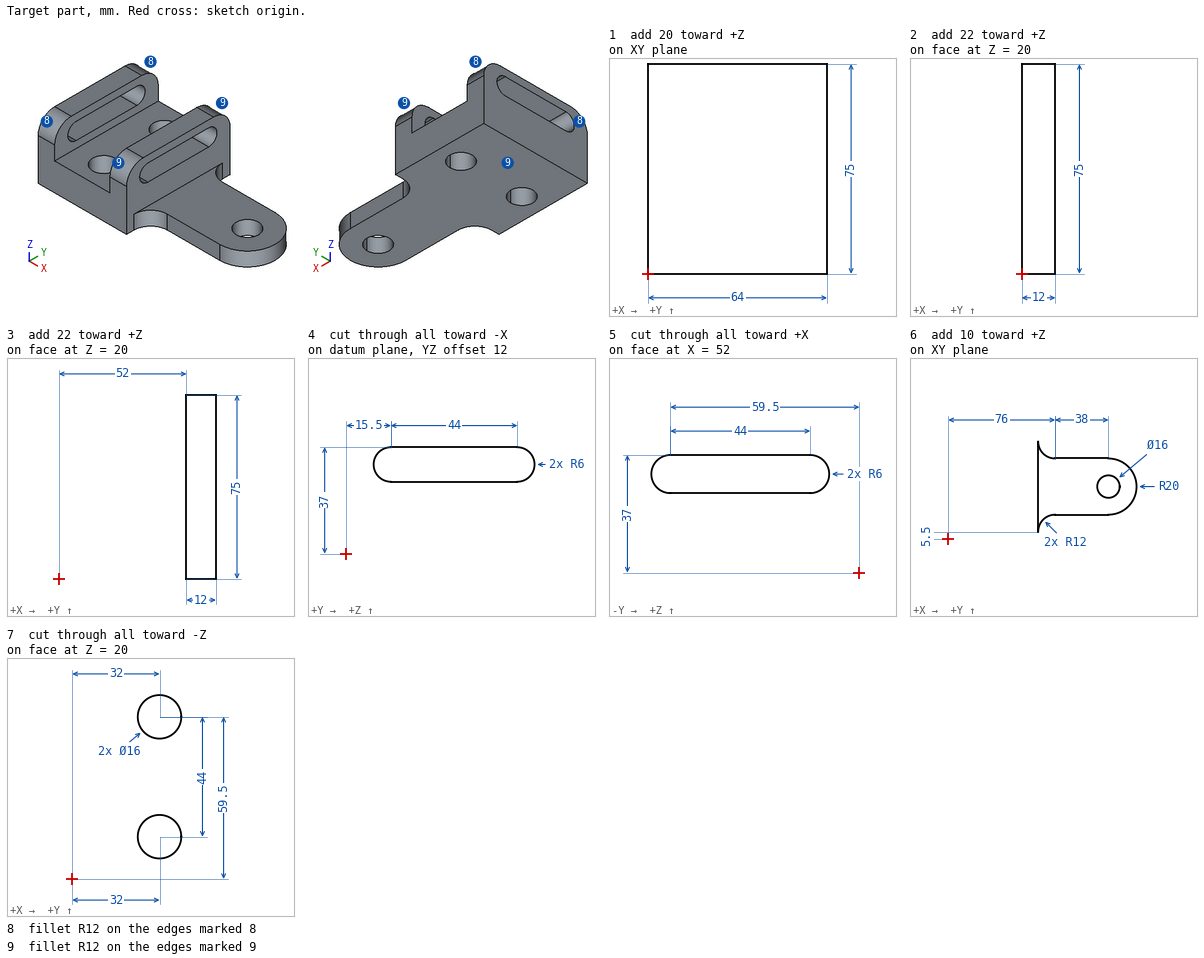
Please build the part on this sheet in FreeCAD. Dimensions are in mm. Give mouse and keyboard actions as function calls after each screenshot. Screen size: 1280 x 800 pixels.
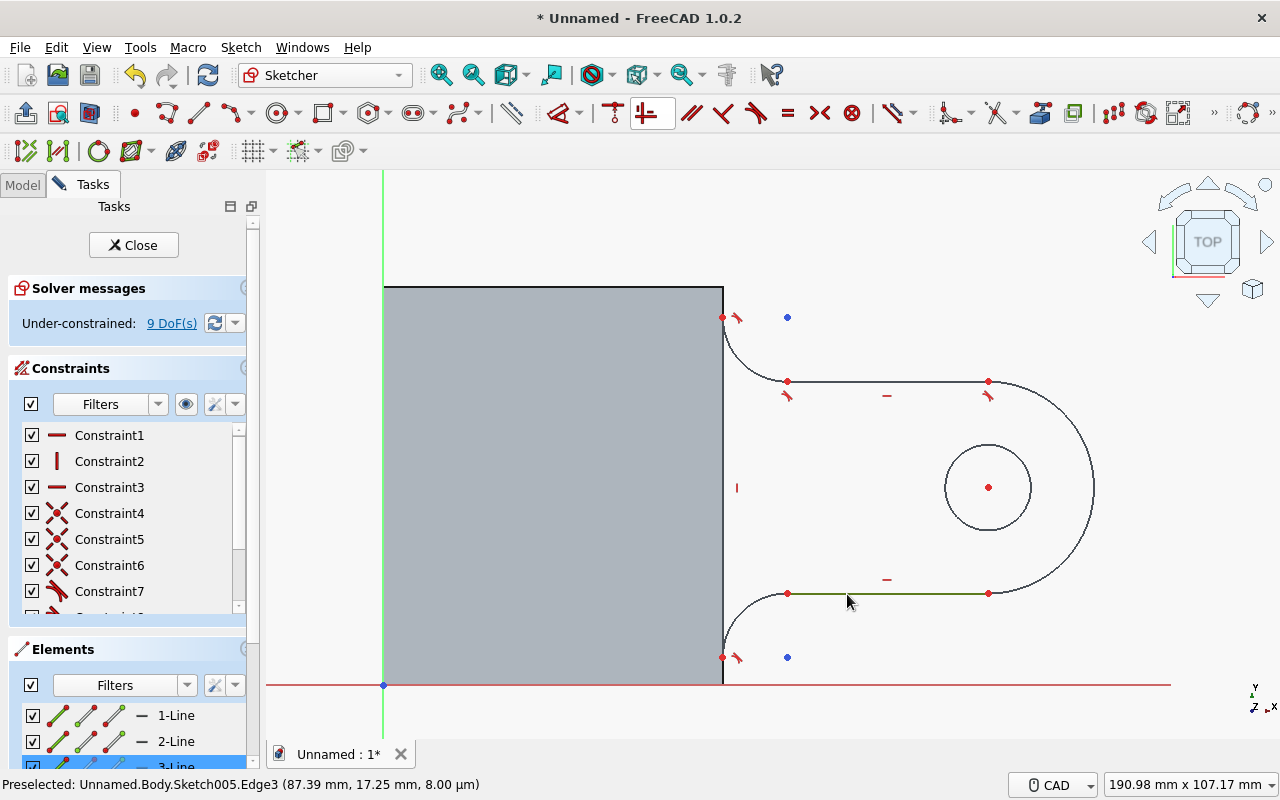
click(758, 601)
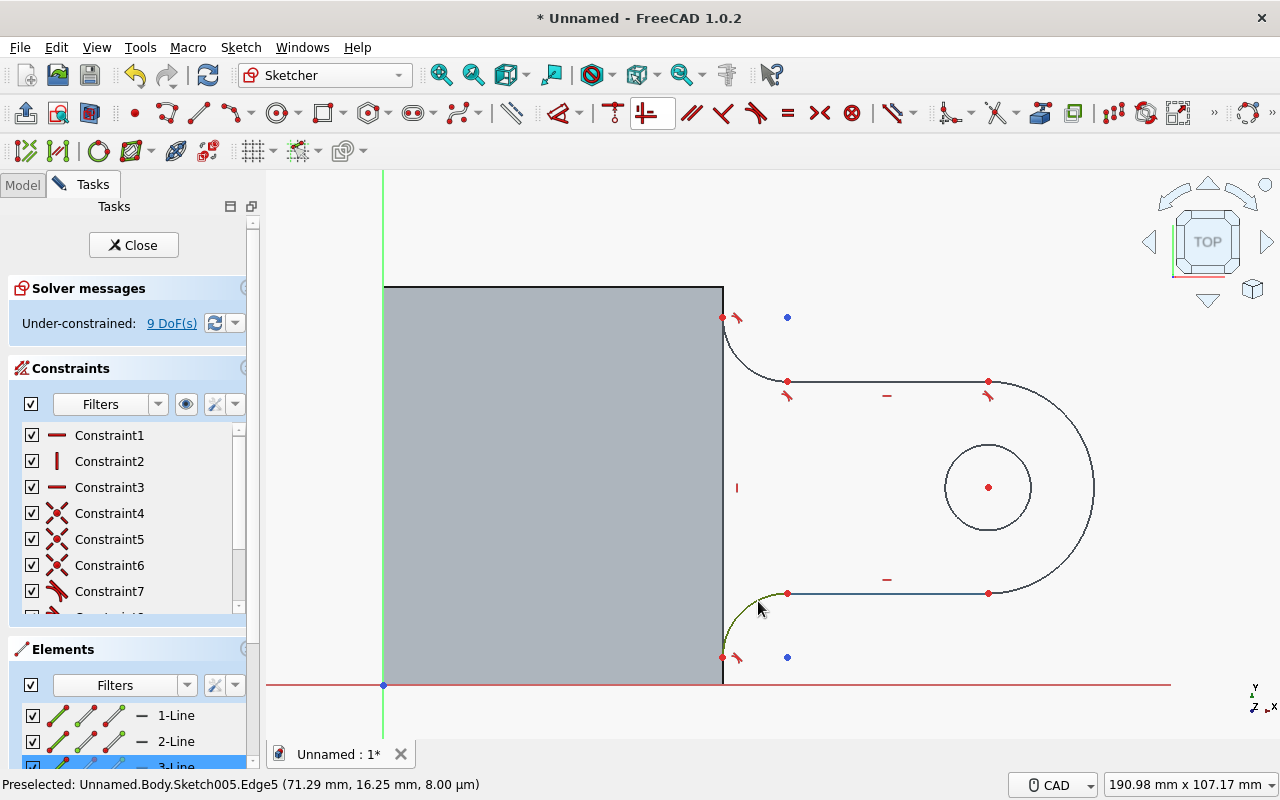
click(756, 114)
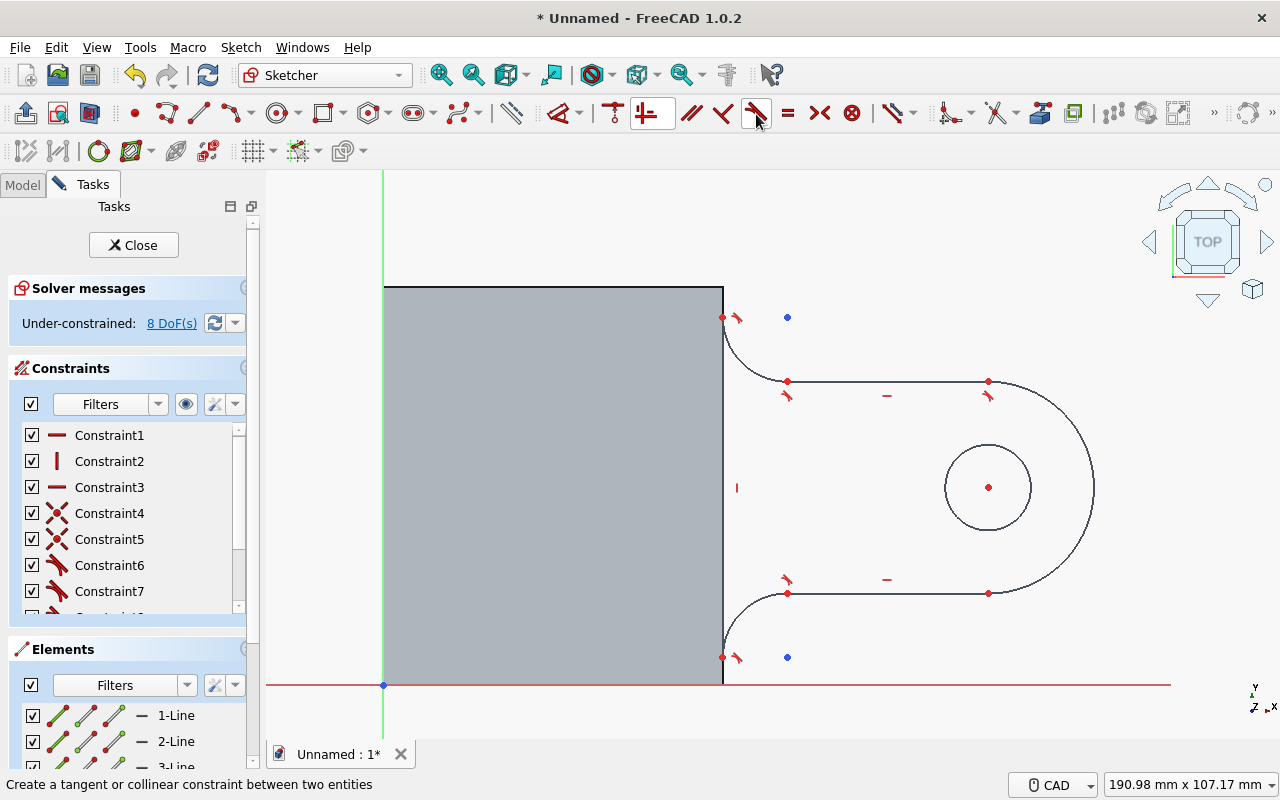
click(847, 594)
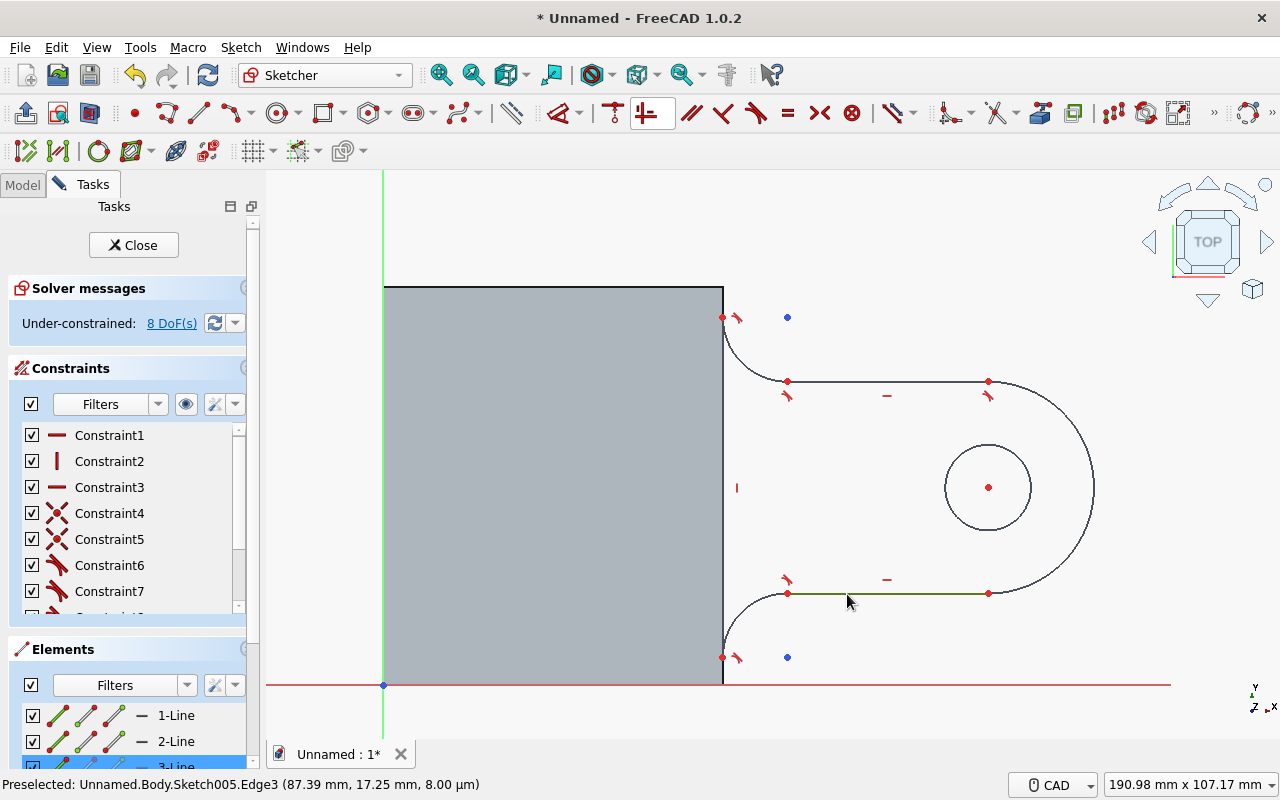
click(1074, 550)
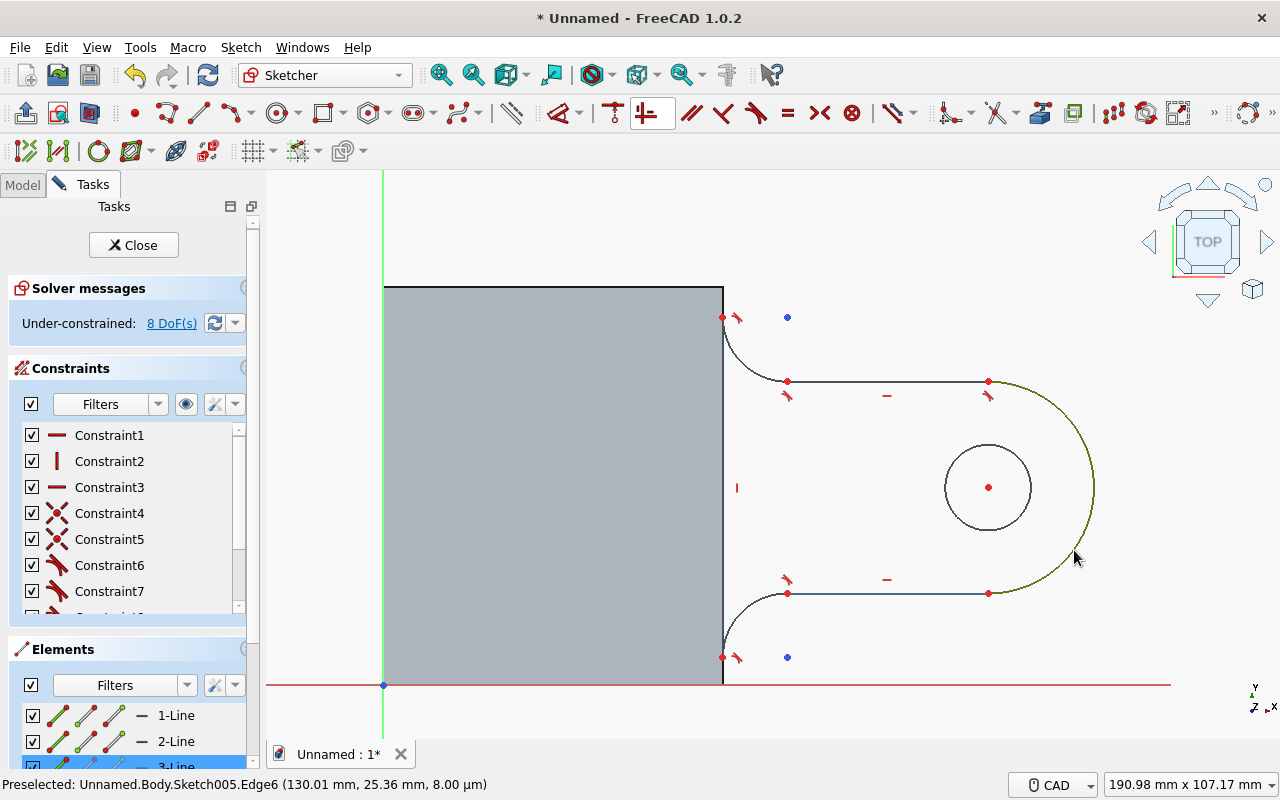
click(756, 114)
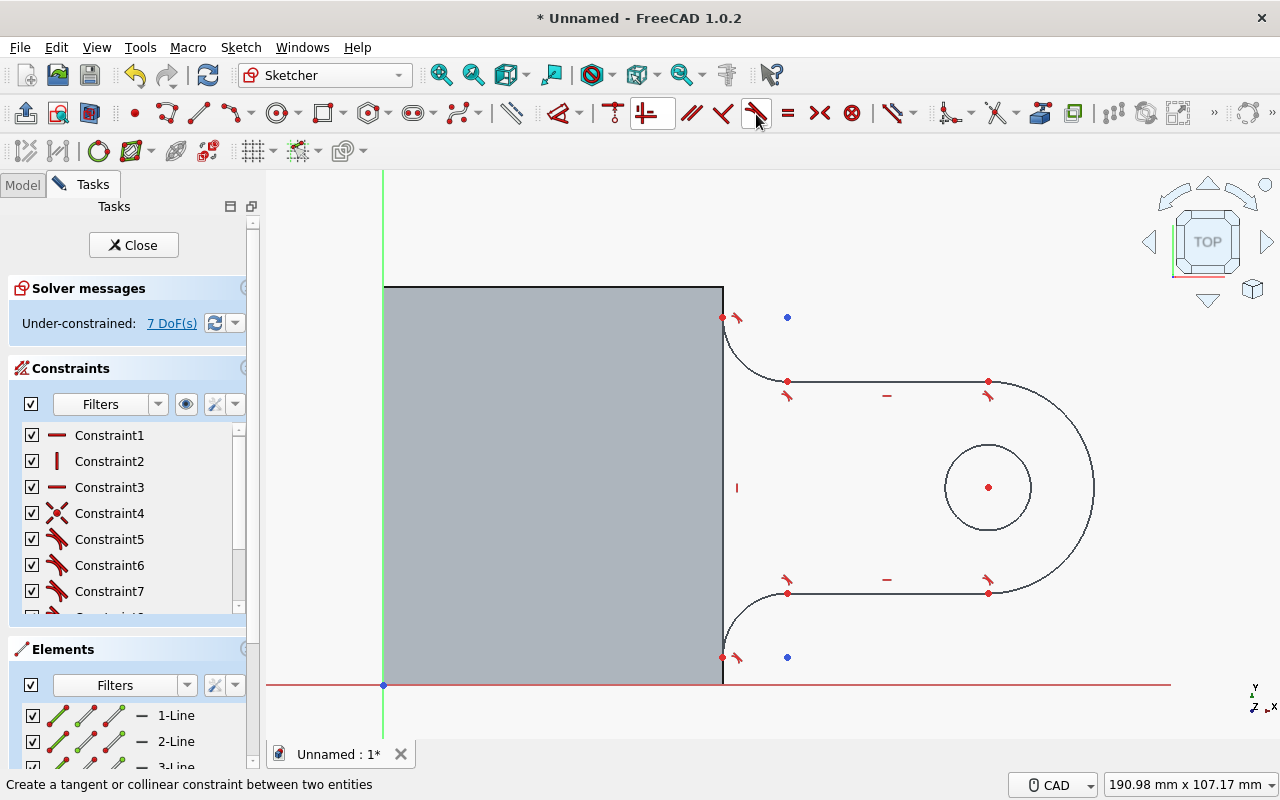
click(758, 375)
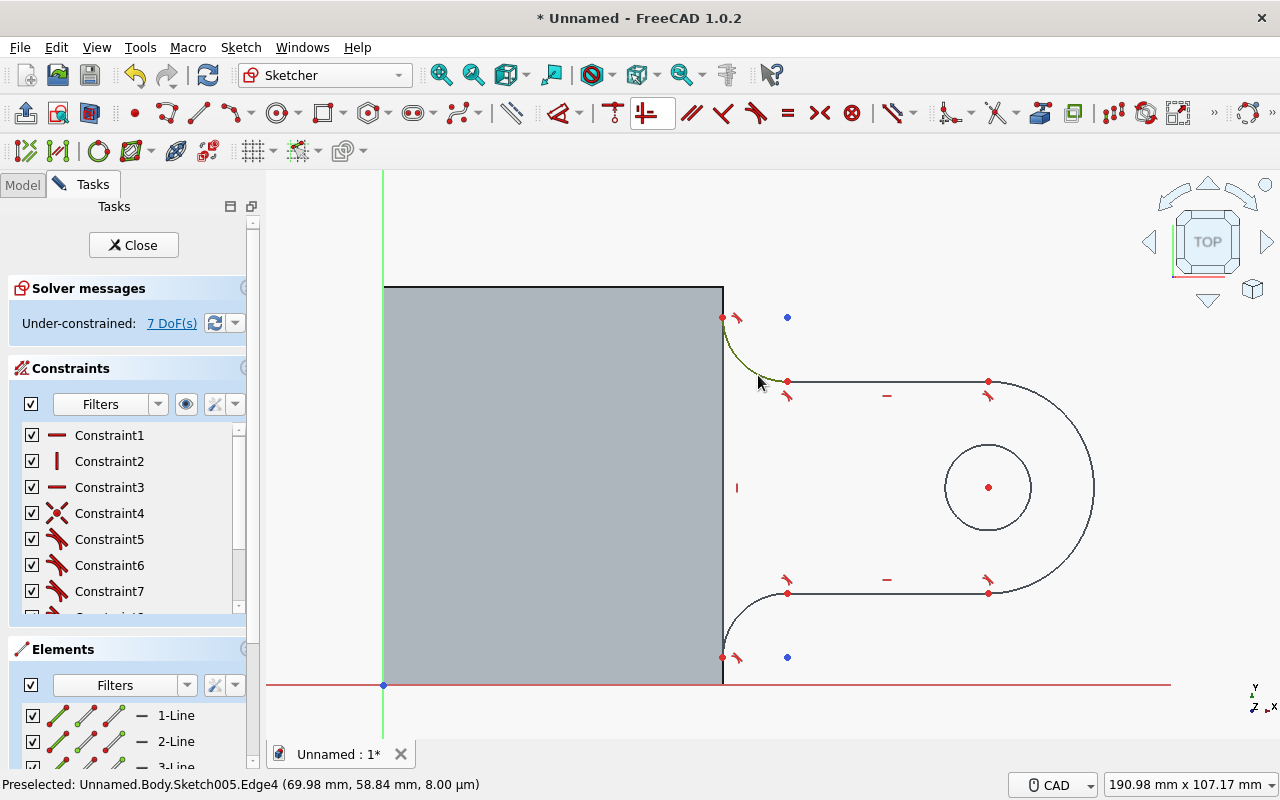
click(758, 601)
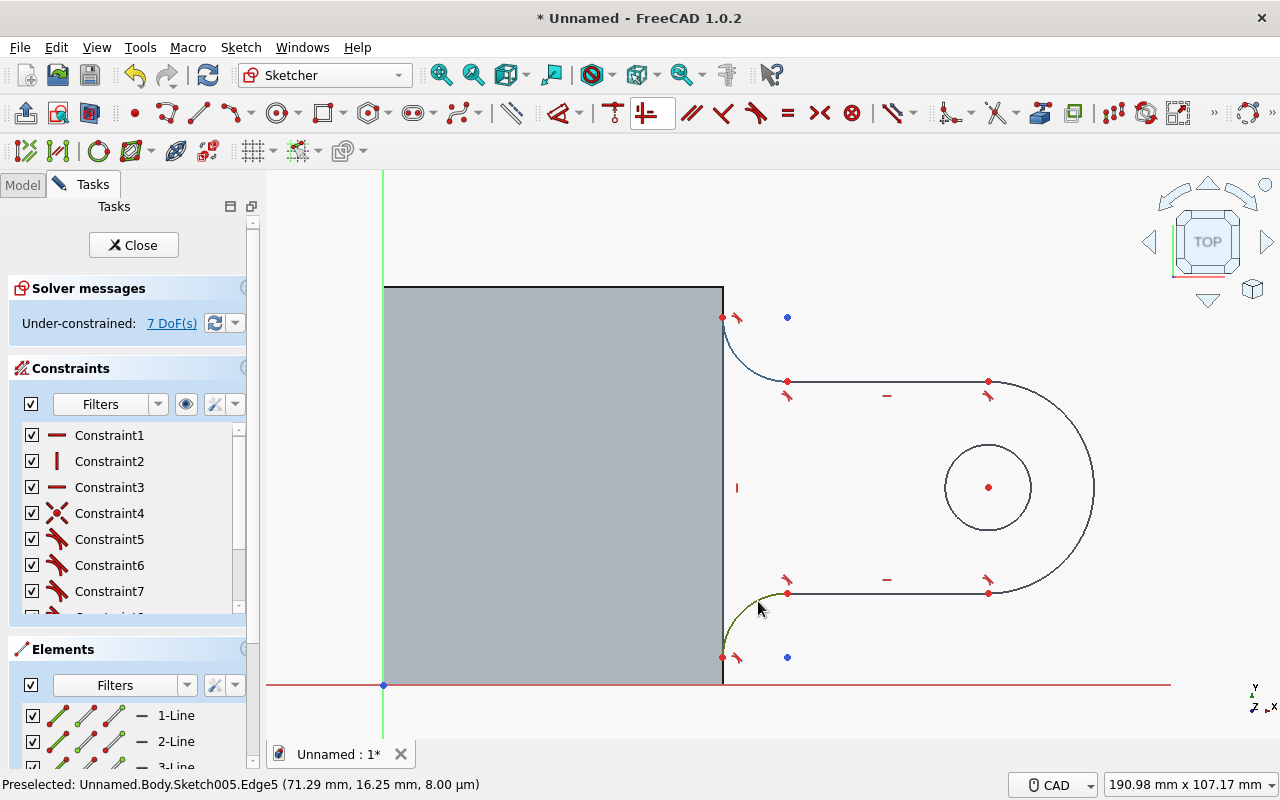
click(788, 114)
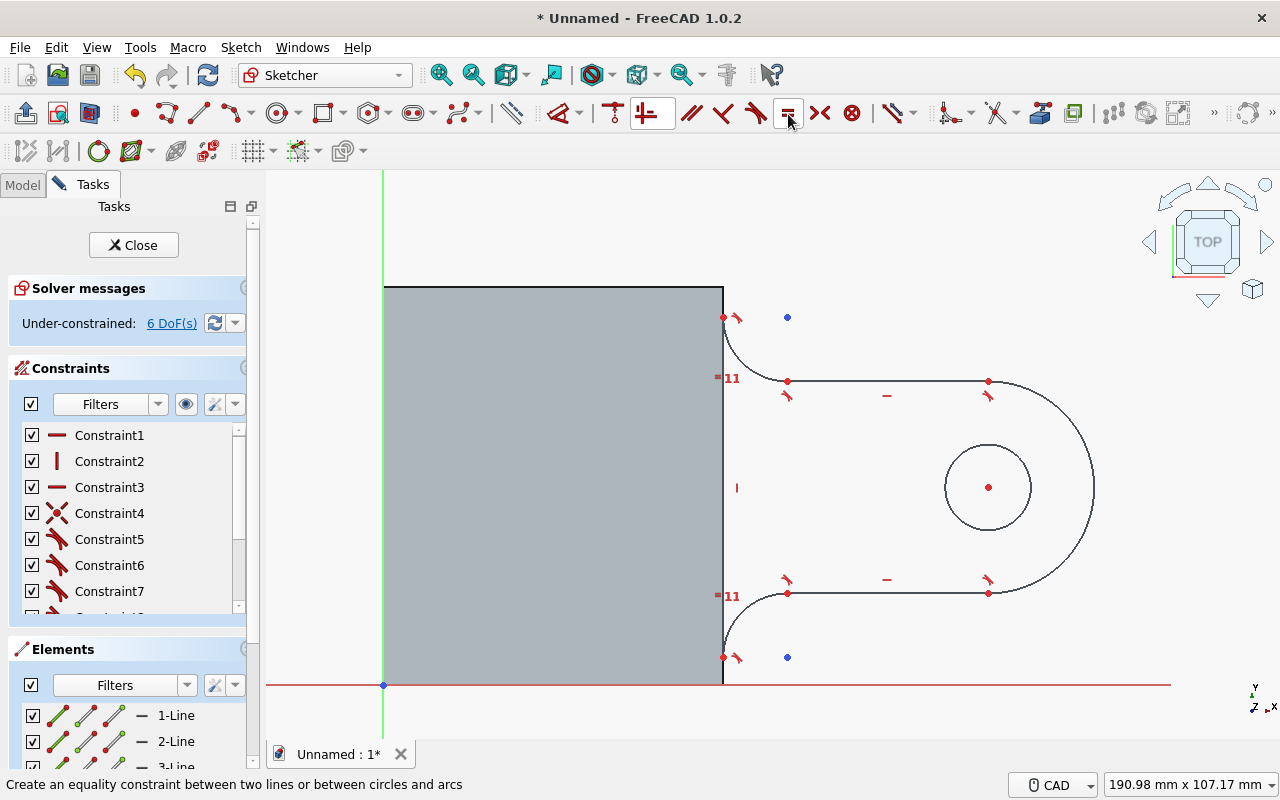
click(558, 114)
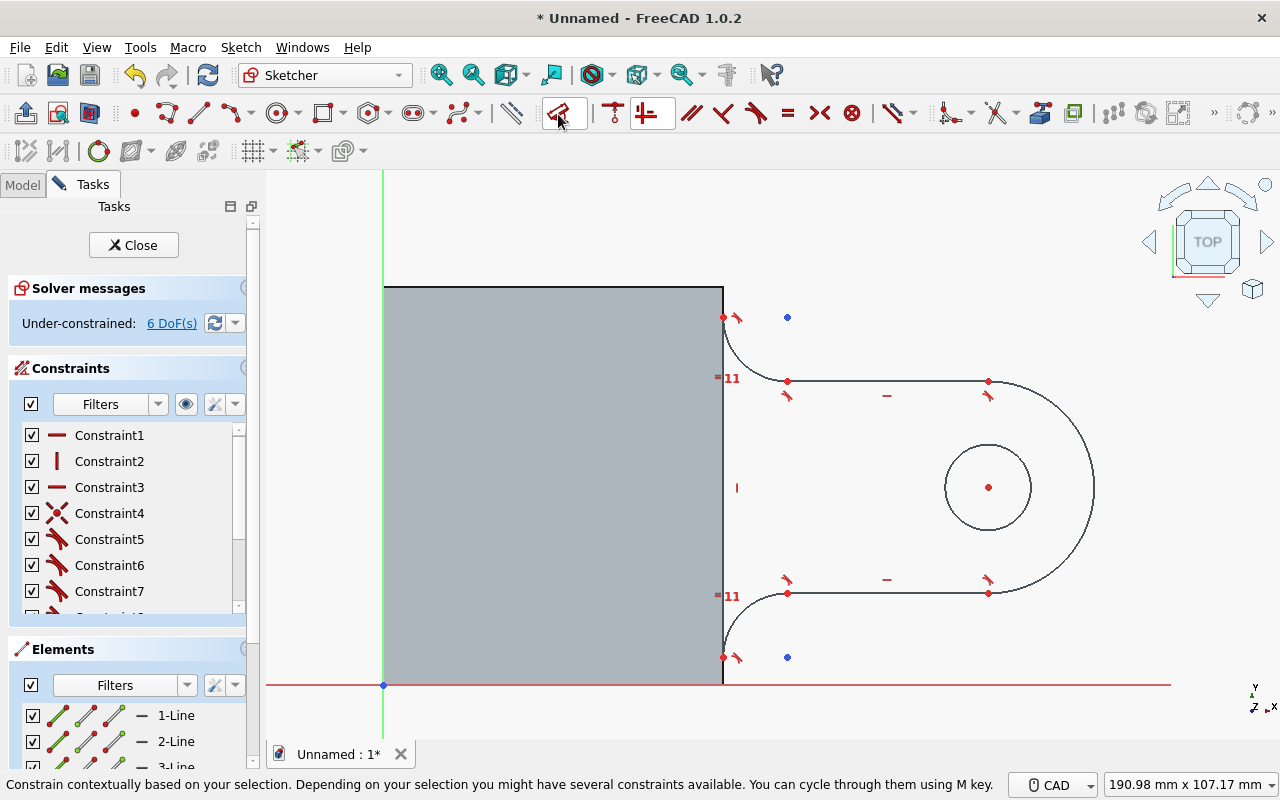
click(758, 374)
click(743, 402)